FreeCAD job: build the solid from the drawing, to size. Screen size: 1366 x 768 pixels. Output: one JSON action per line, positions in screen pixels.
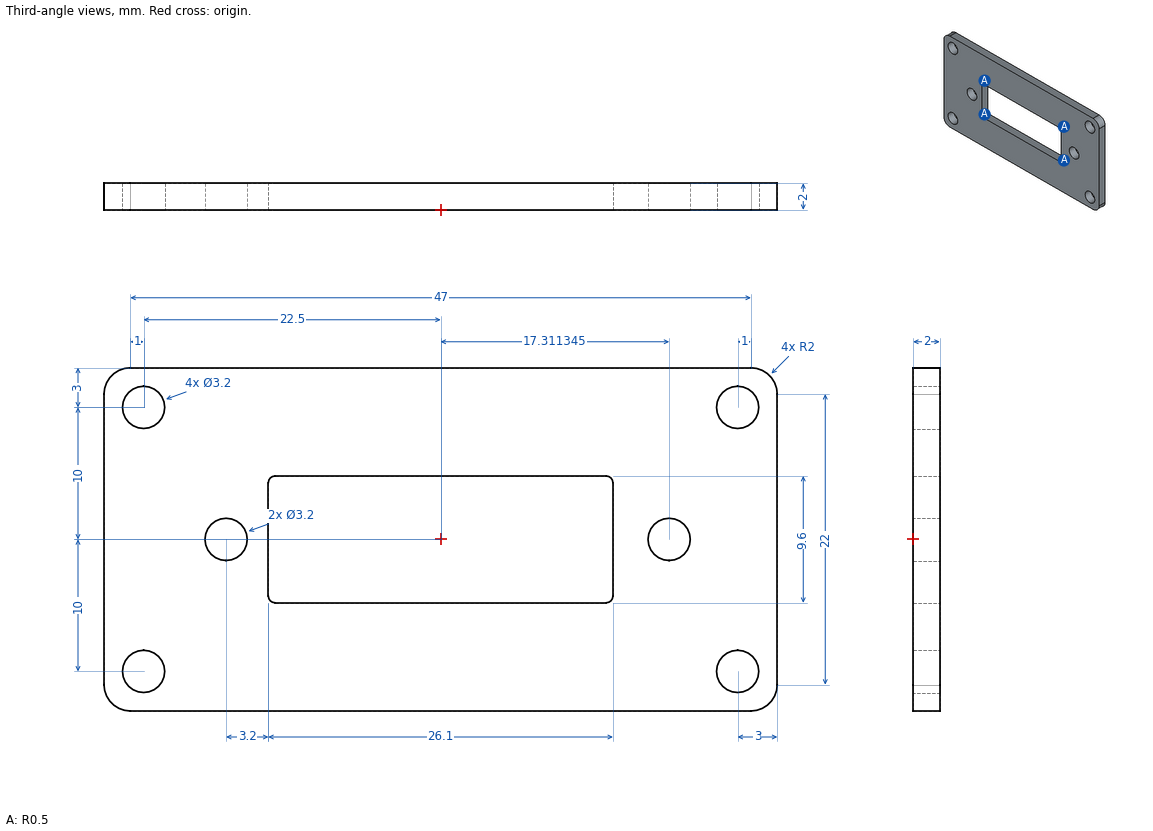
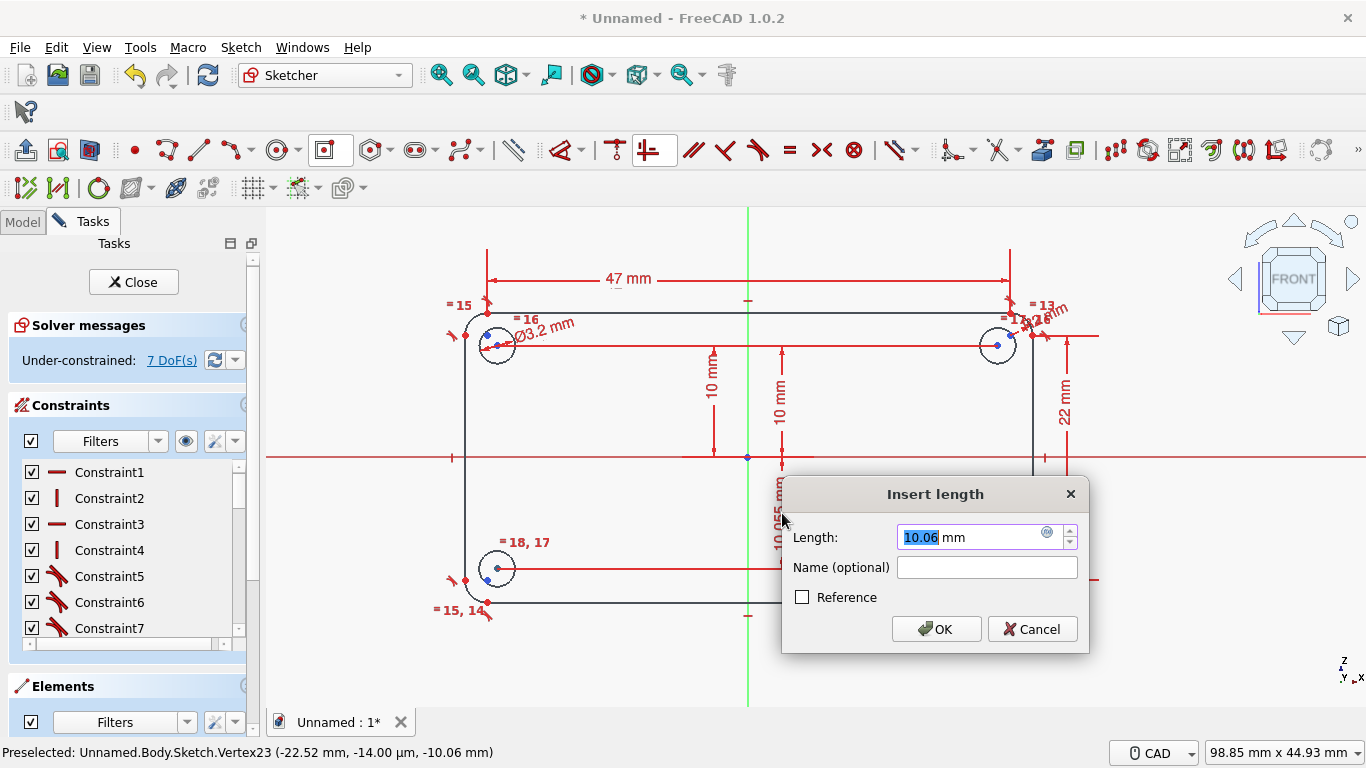
{"action": "type", "text": "10"}
{"action": "key", "text": "Return"}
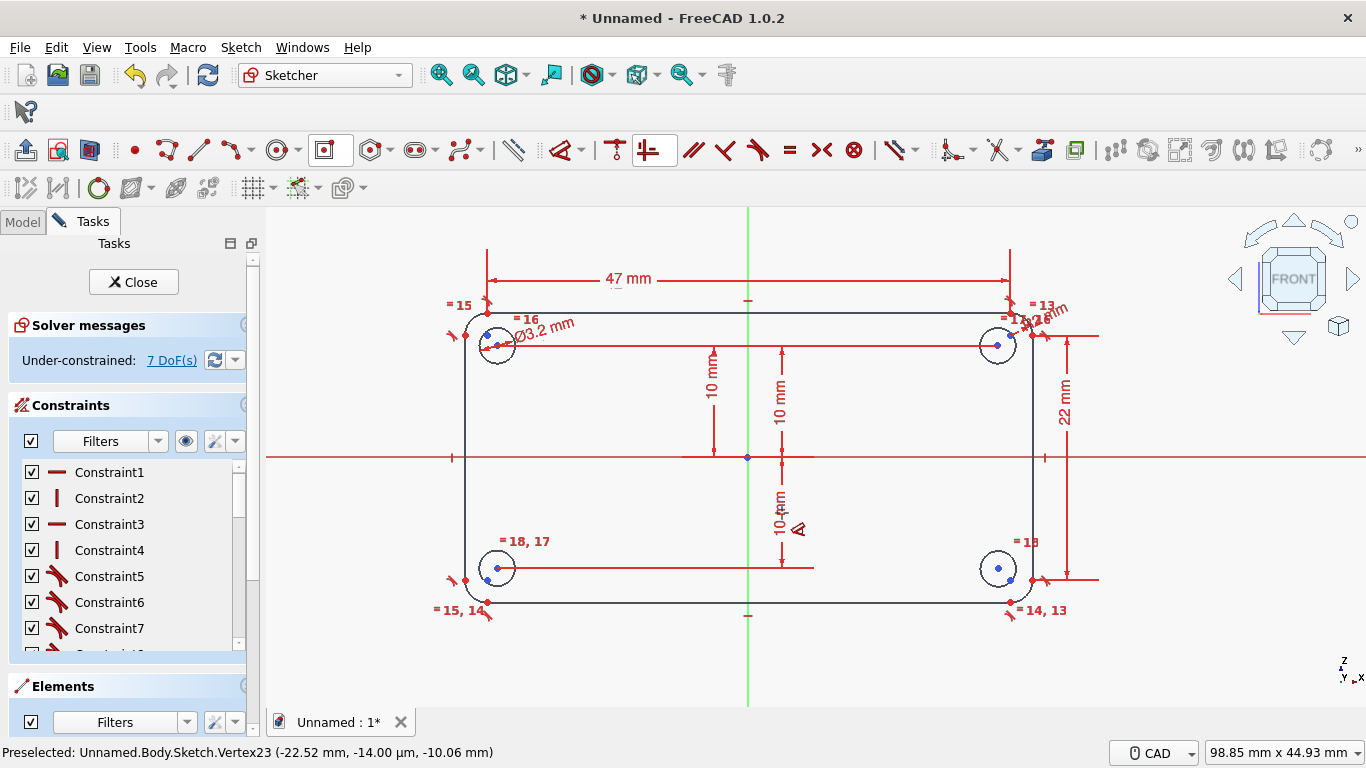
{"action": "left_click", "coordinate": [998, 569]}
{"action": "left_click", "coordinate": [714, 487]}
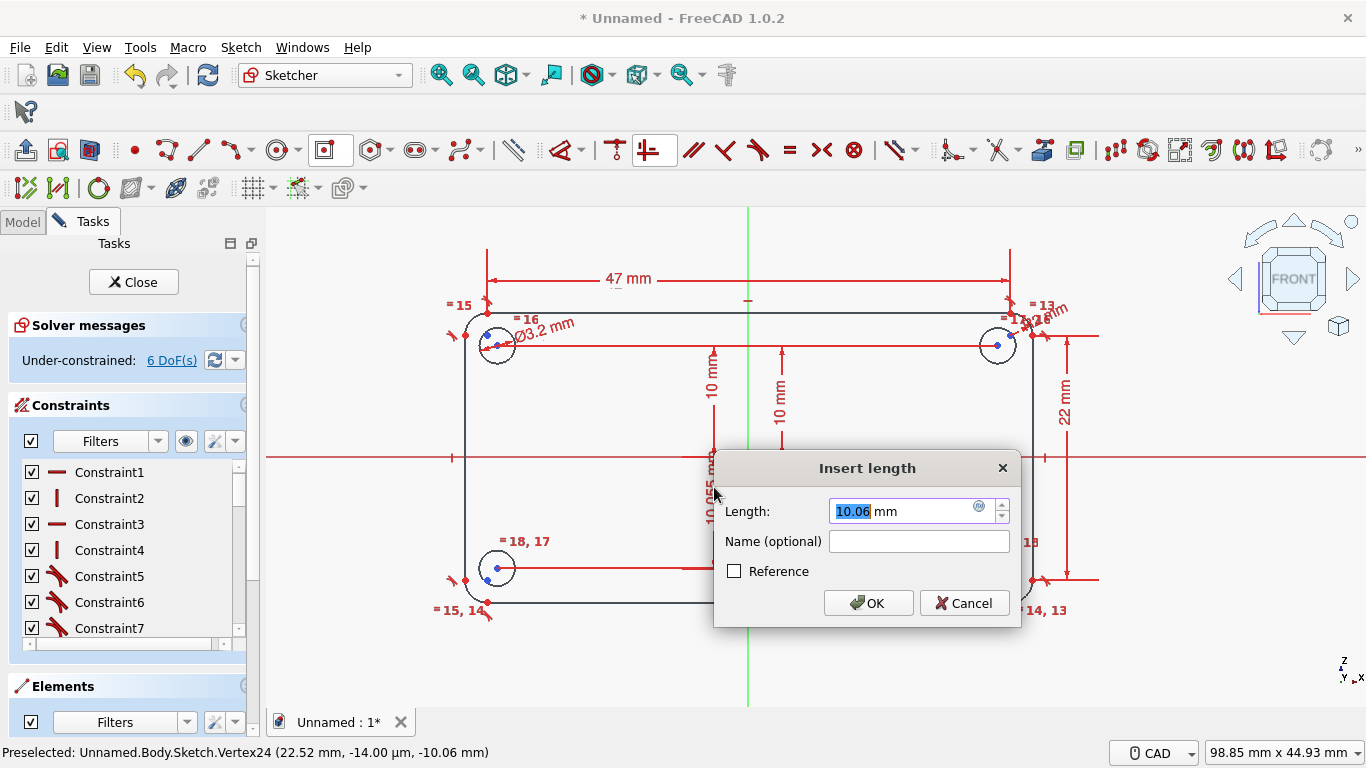
{"action": "type", "text": "10"}
{"action": "key", "text": "Return"}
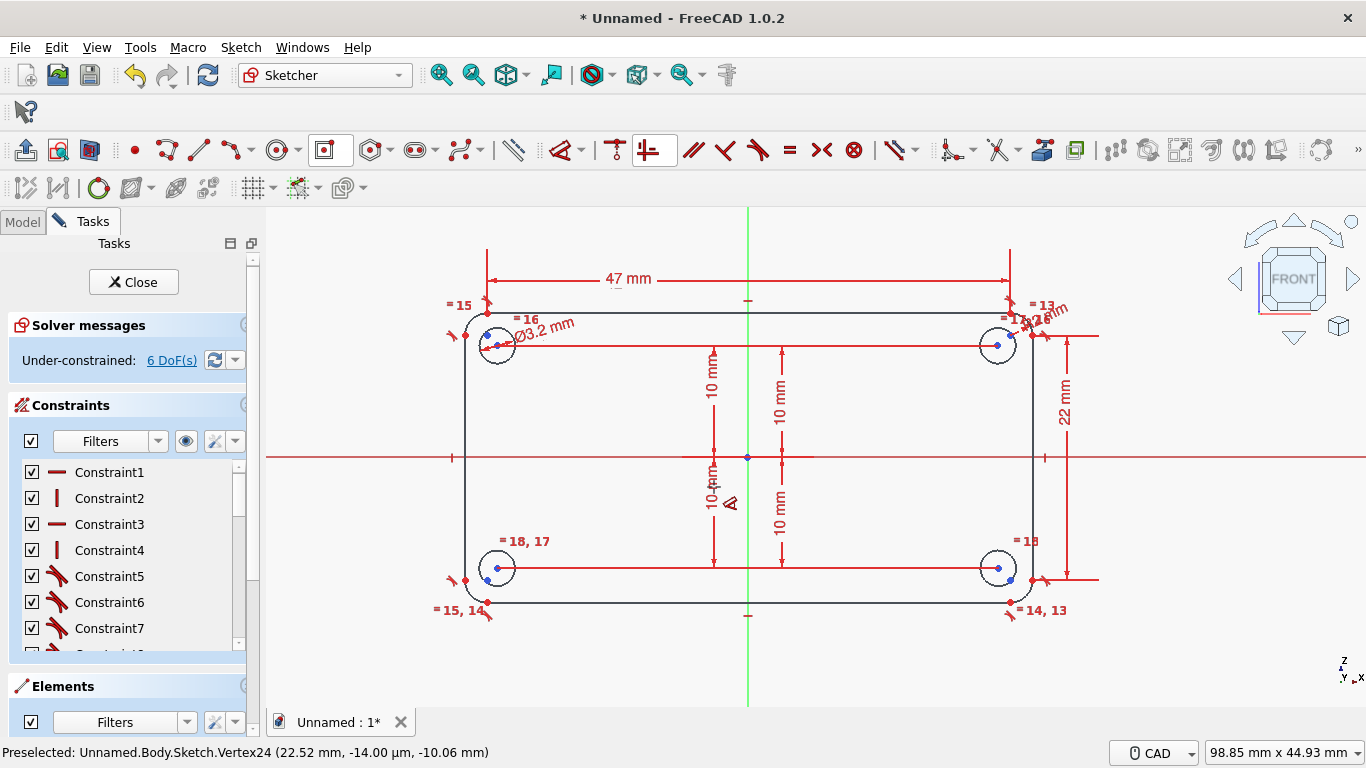
{"action": "scroll", "coordinate": [487, 313], "scroll_direction": "up", "scroll_amount": 7}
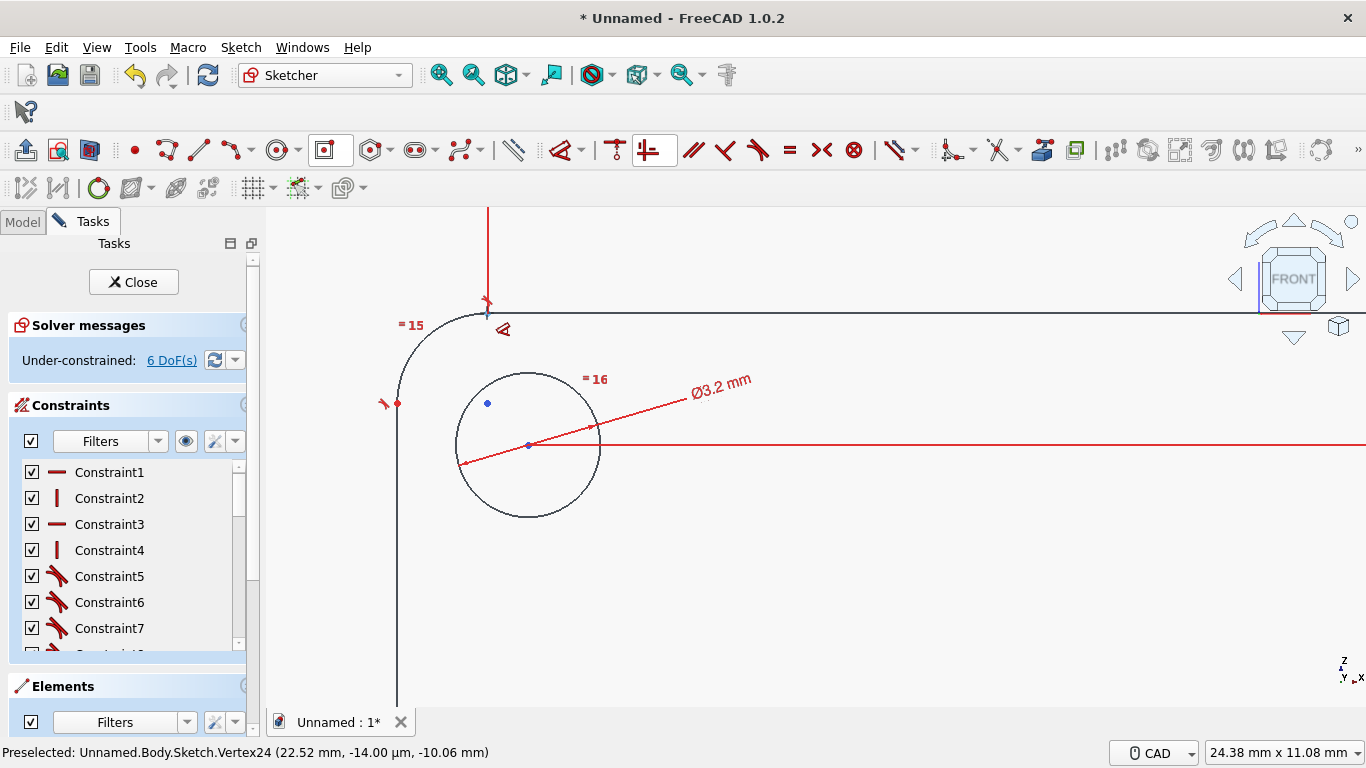
{"action": "left_click", "coordinate": [488, 313]}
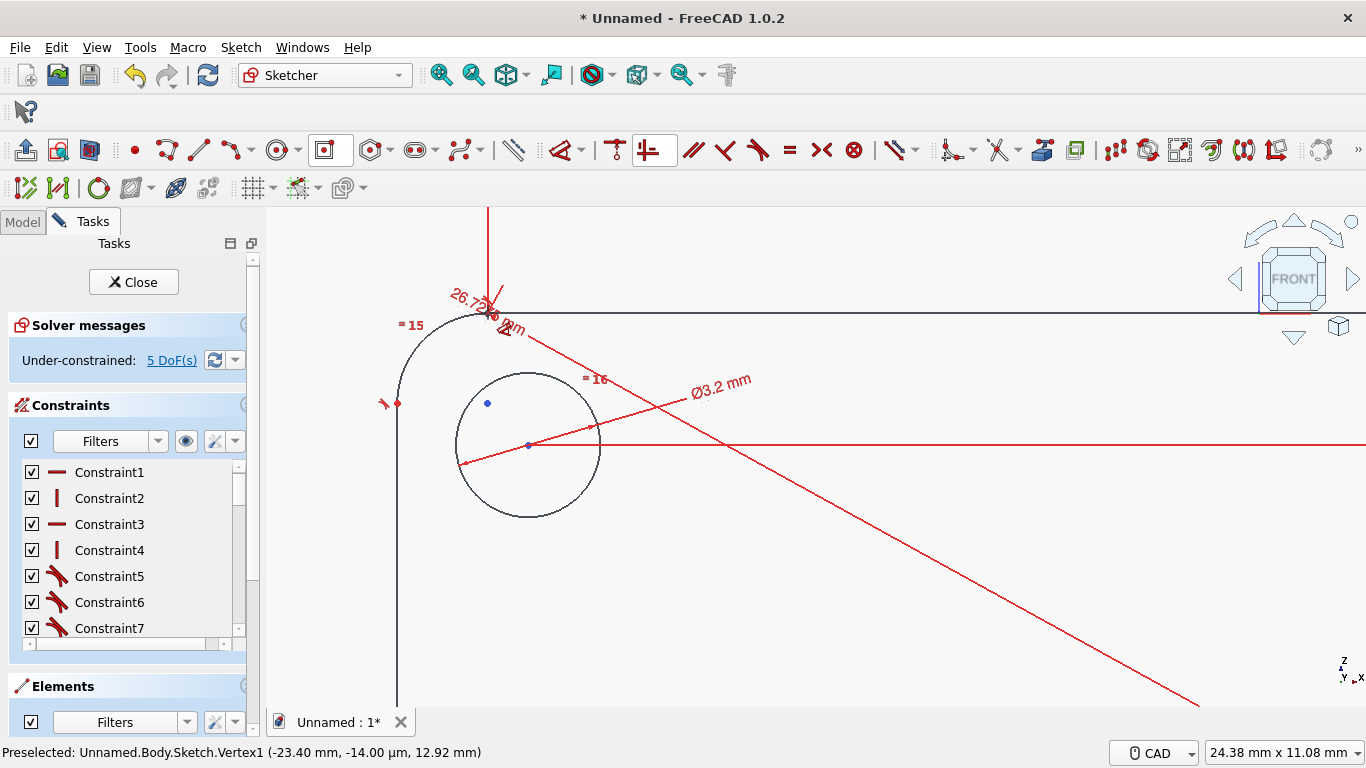
{"action": "left_click", "coordinate": [528, 445]}
{"action": "left_click", "coordinate": [508, 279]}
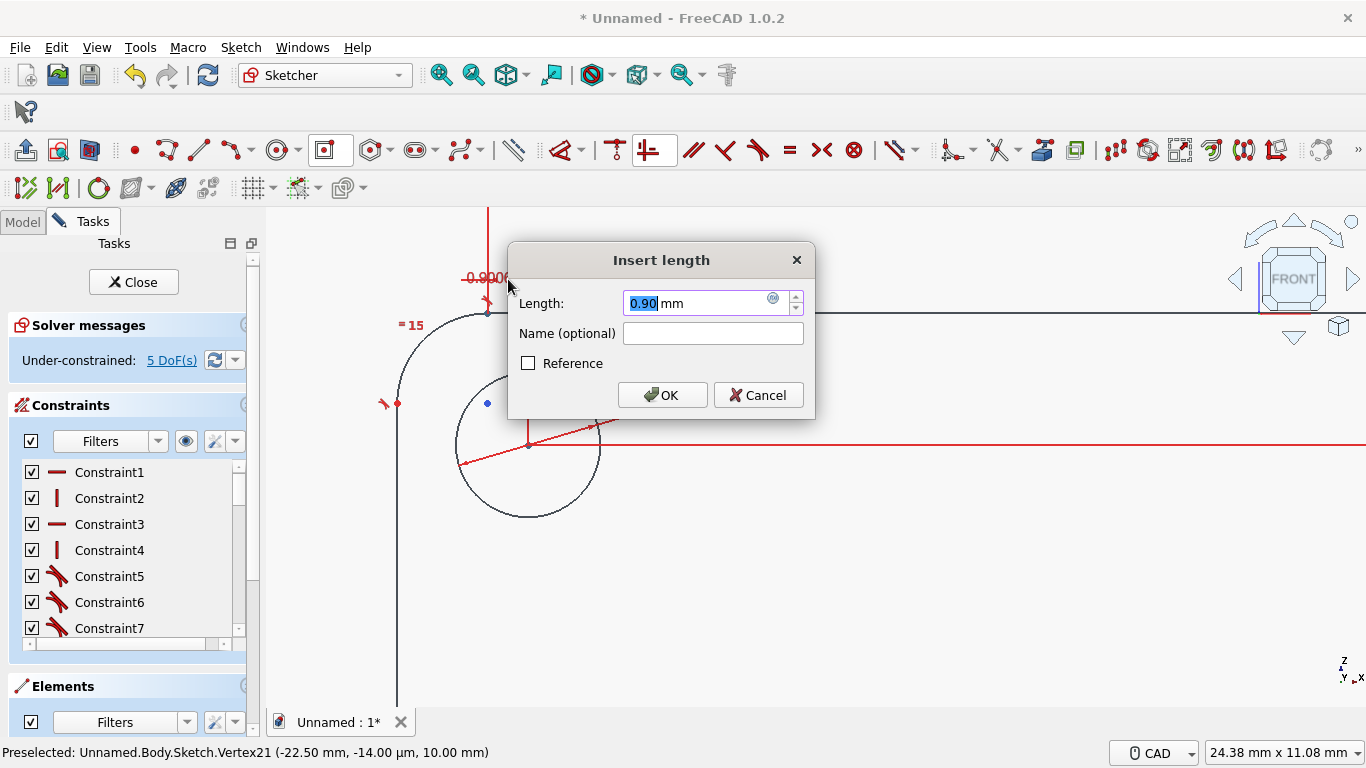
{"action": "type", "text": "1"}
{"action": "key", "text": "Return"}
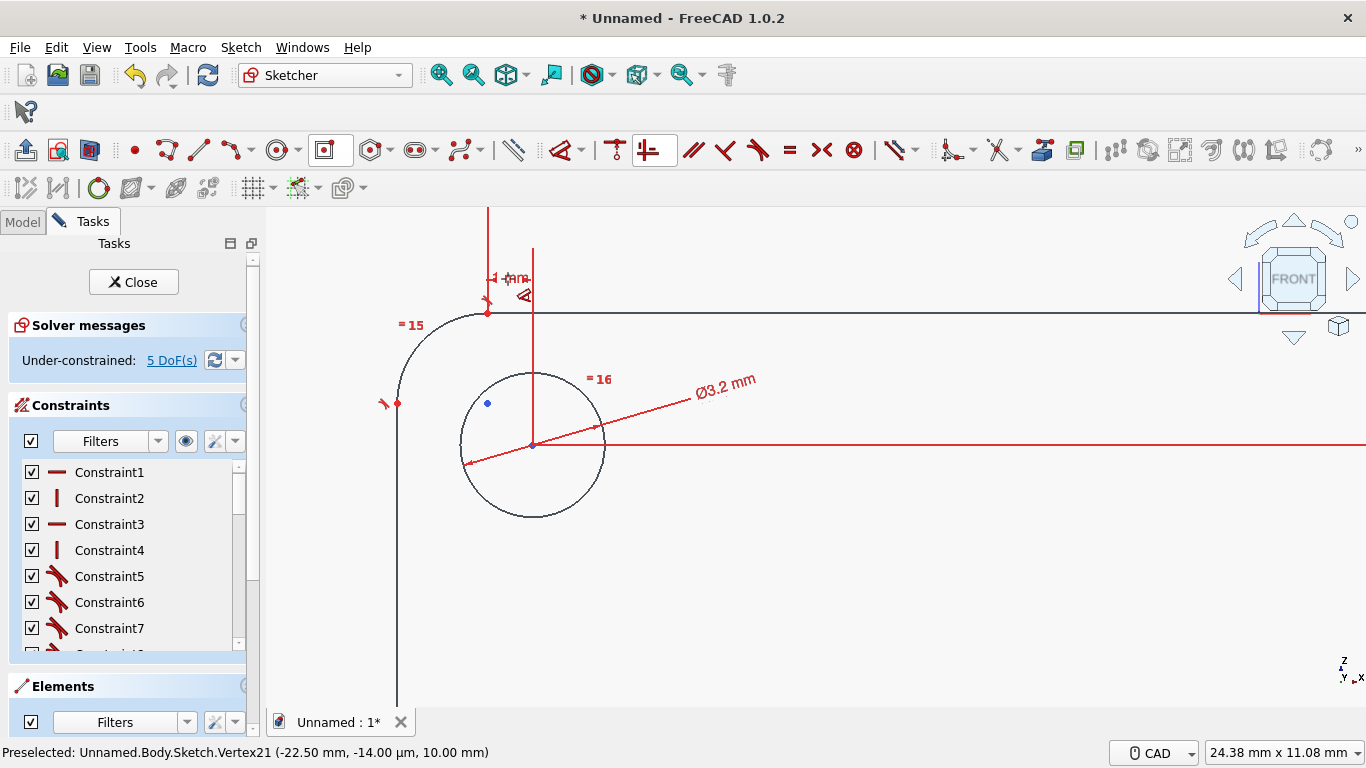
{"action": "scroll", "coordinate": [487, 313], "scroll_direction": "down", "scroll_amount": 7}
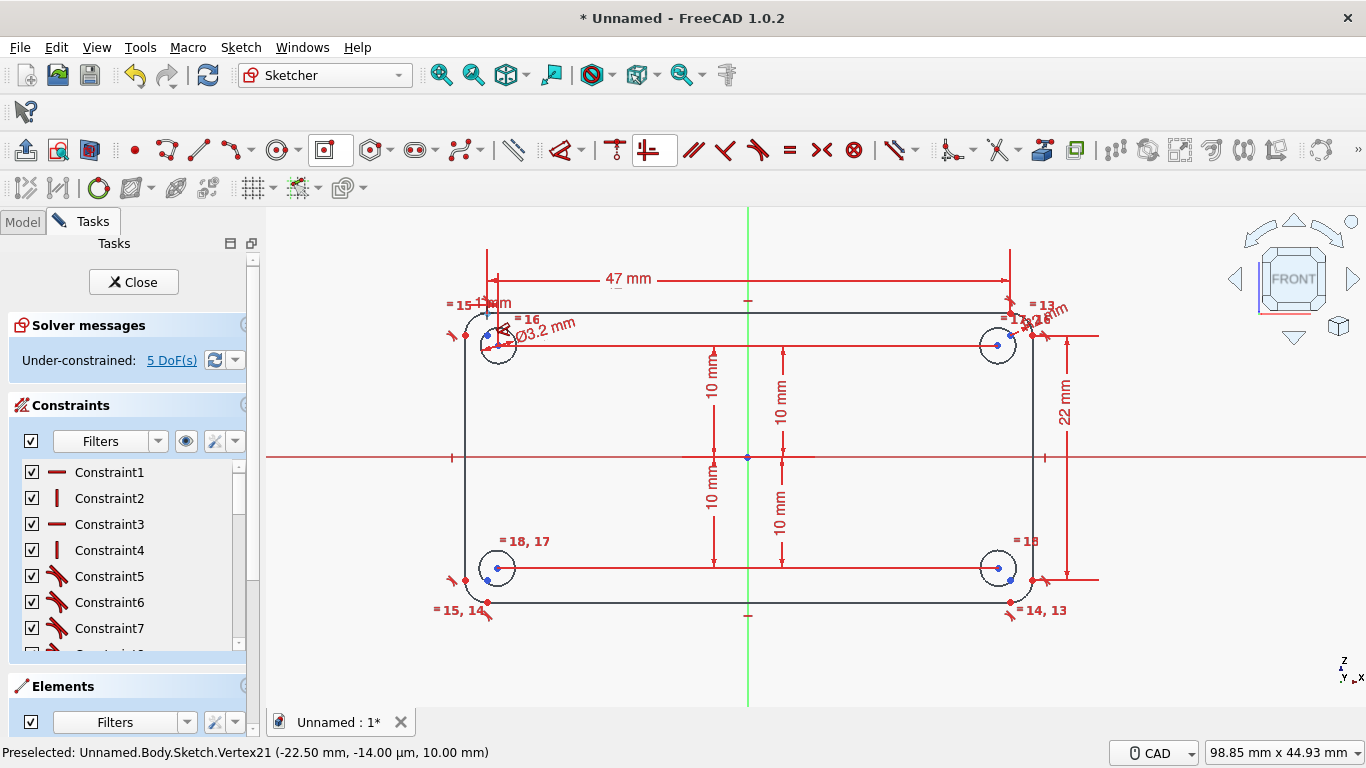
{"action": "left_click", "coordinate": [487, 313]}